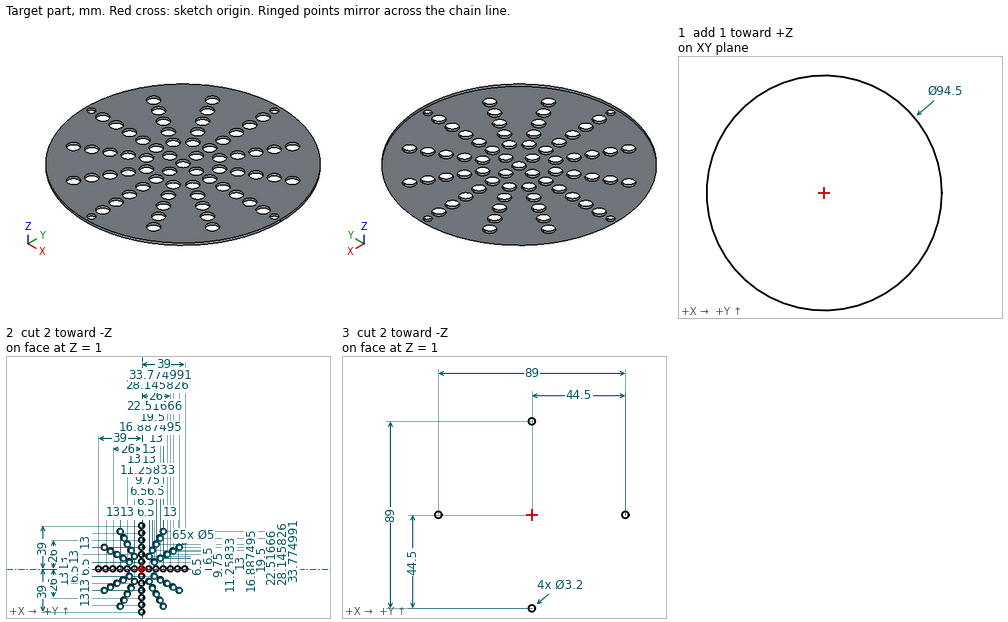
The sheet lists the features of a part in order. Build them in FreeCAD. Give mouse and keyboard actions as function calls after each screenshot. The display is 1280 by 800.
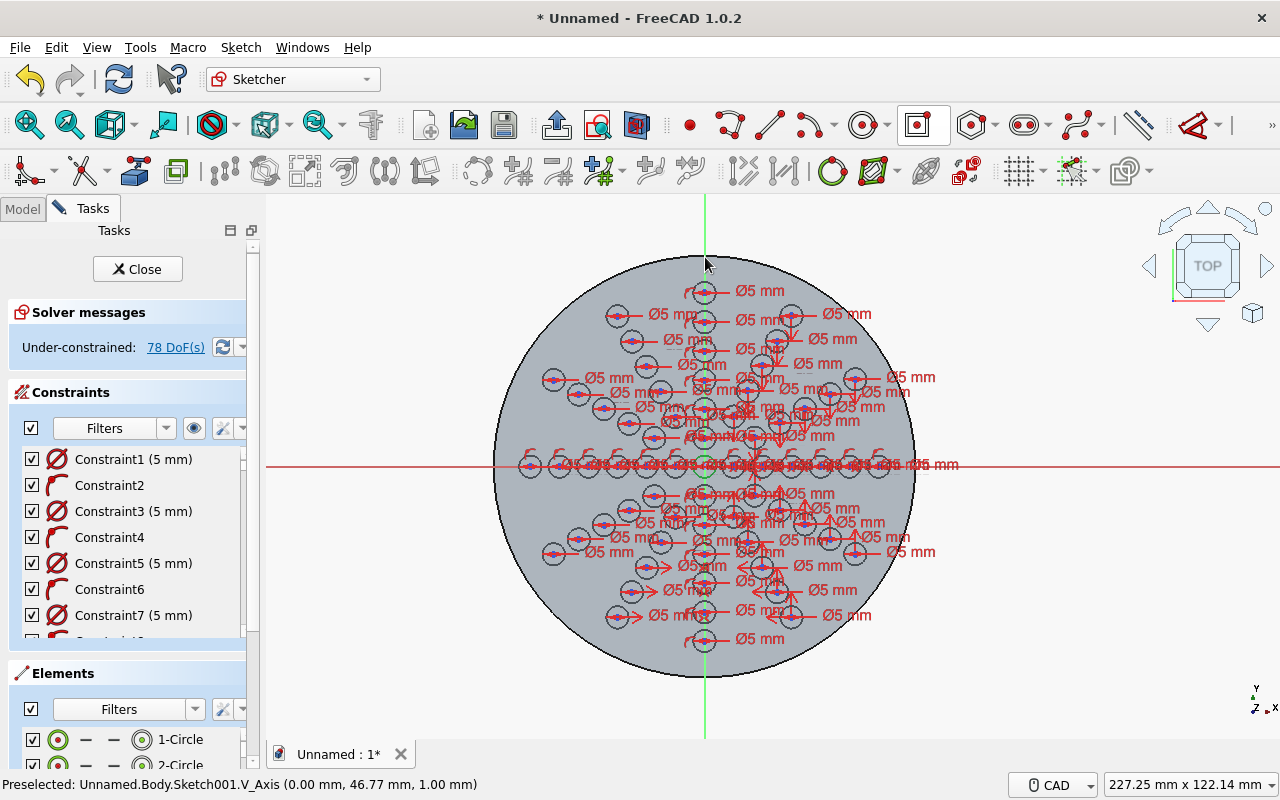
click(748, 542)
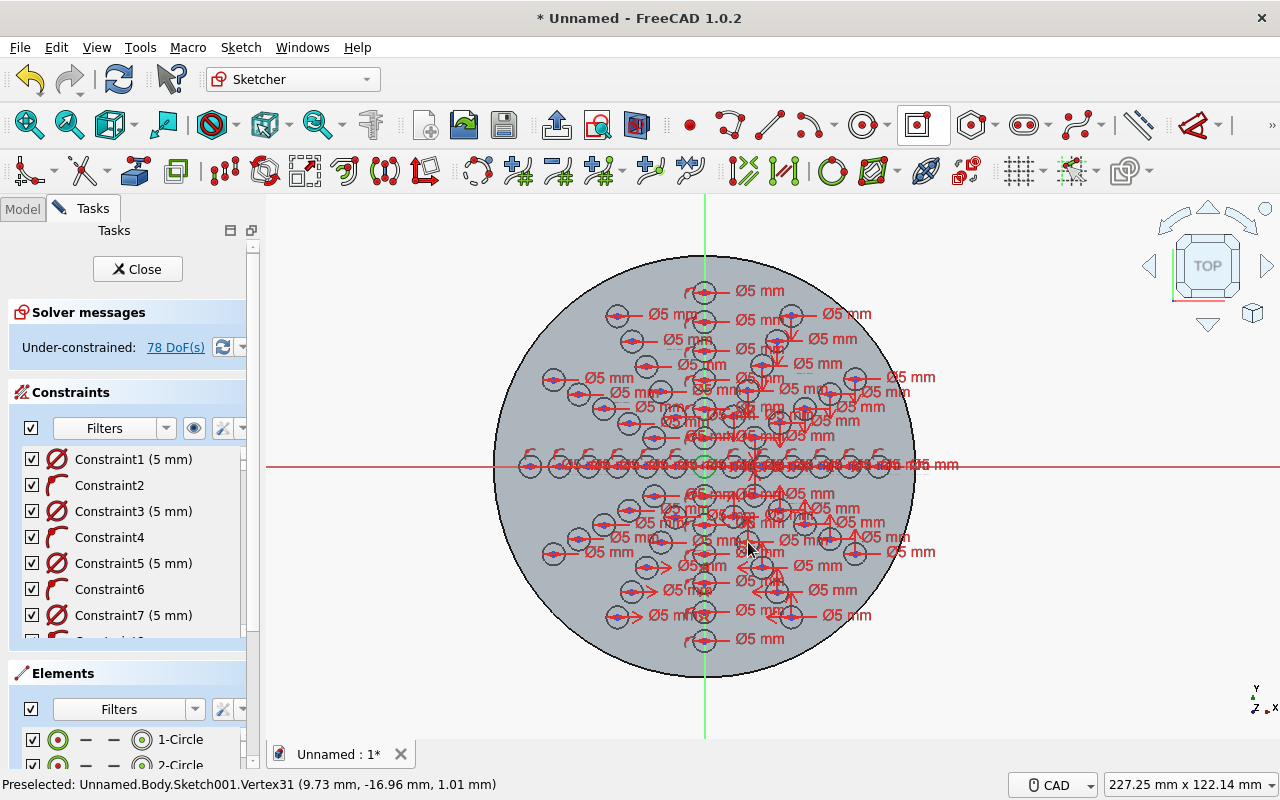
click(661, 543)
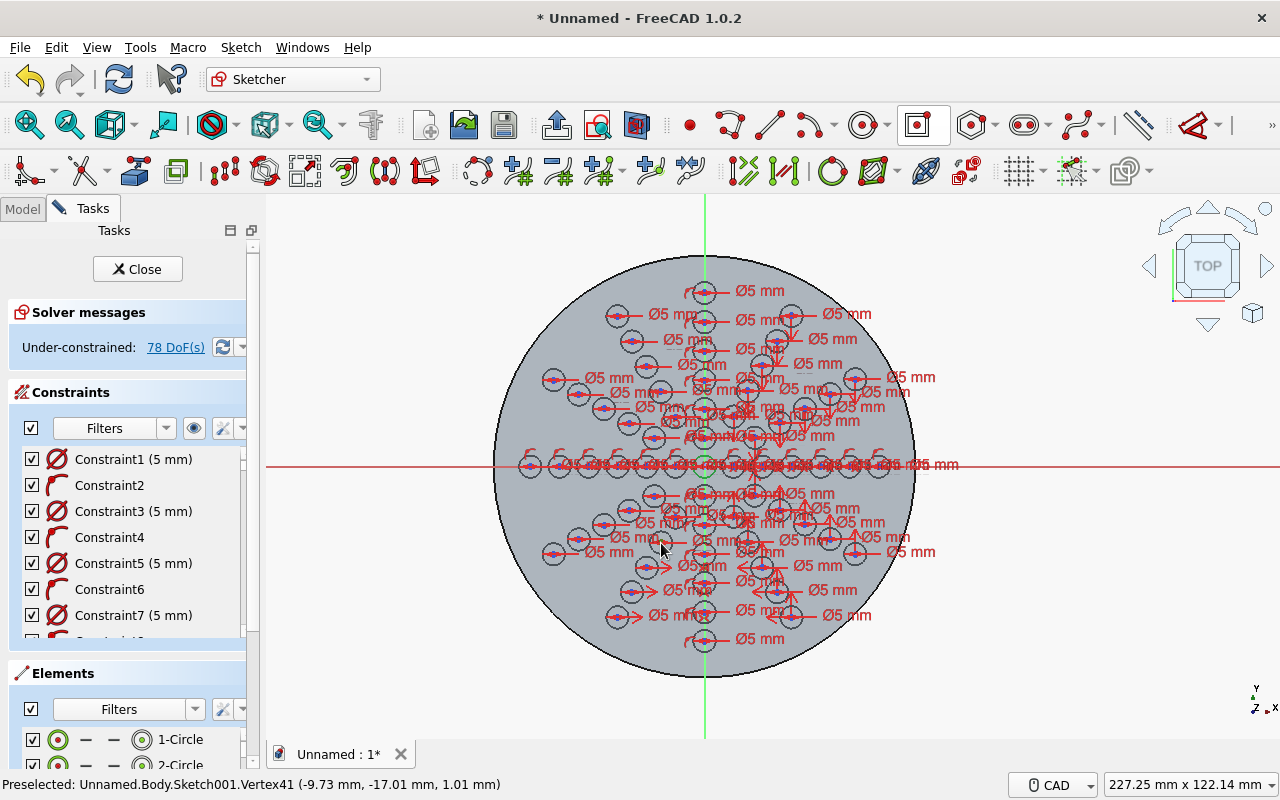
click(705, 257)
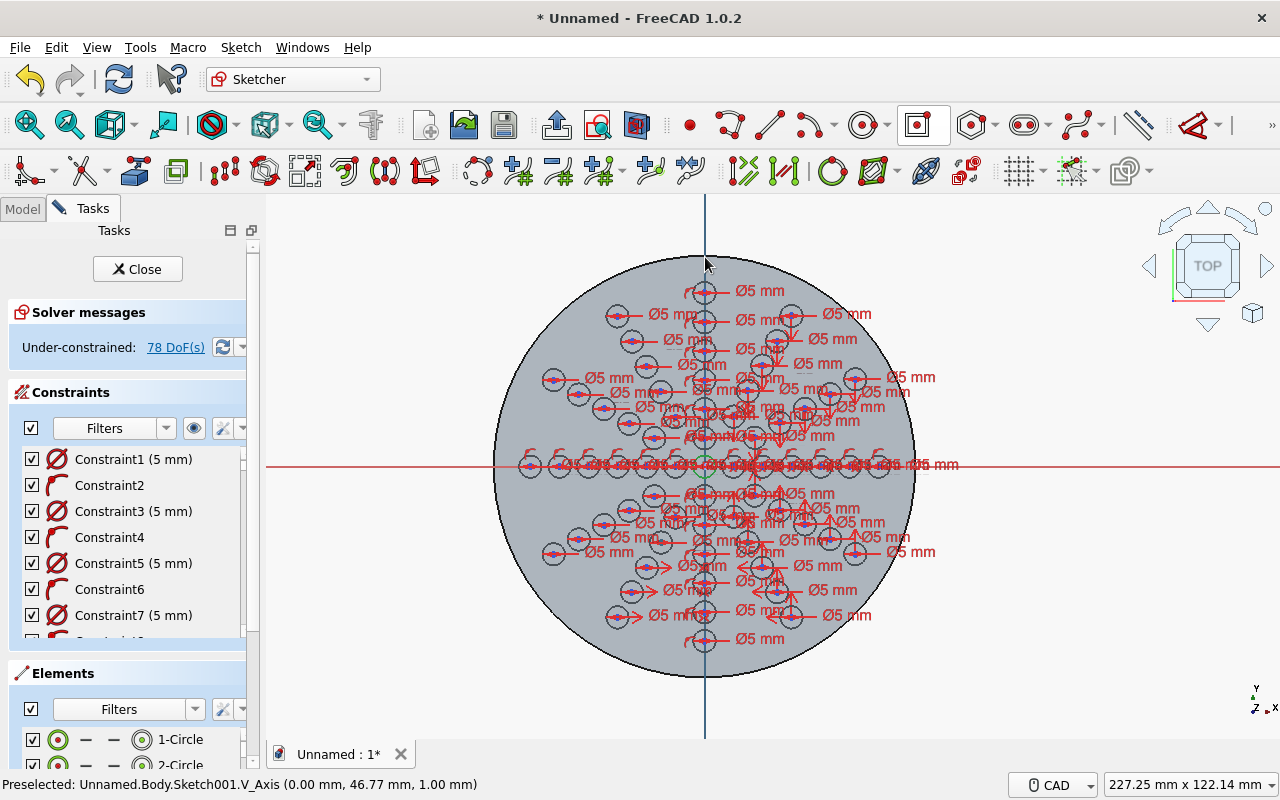
key(s)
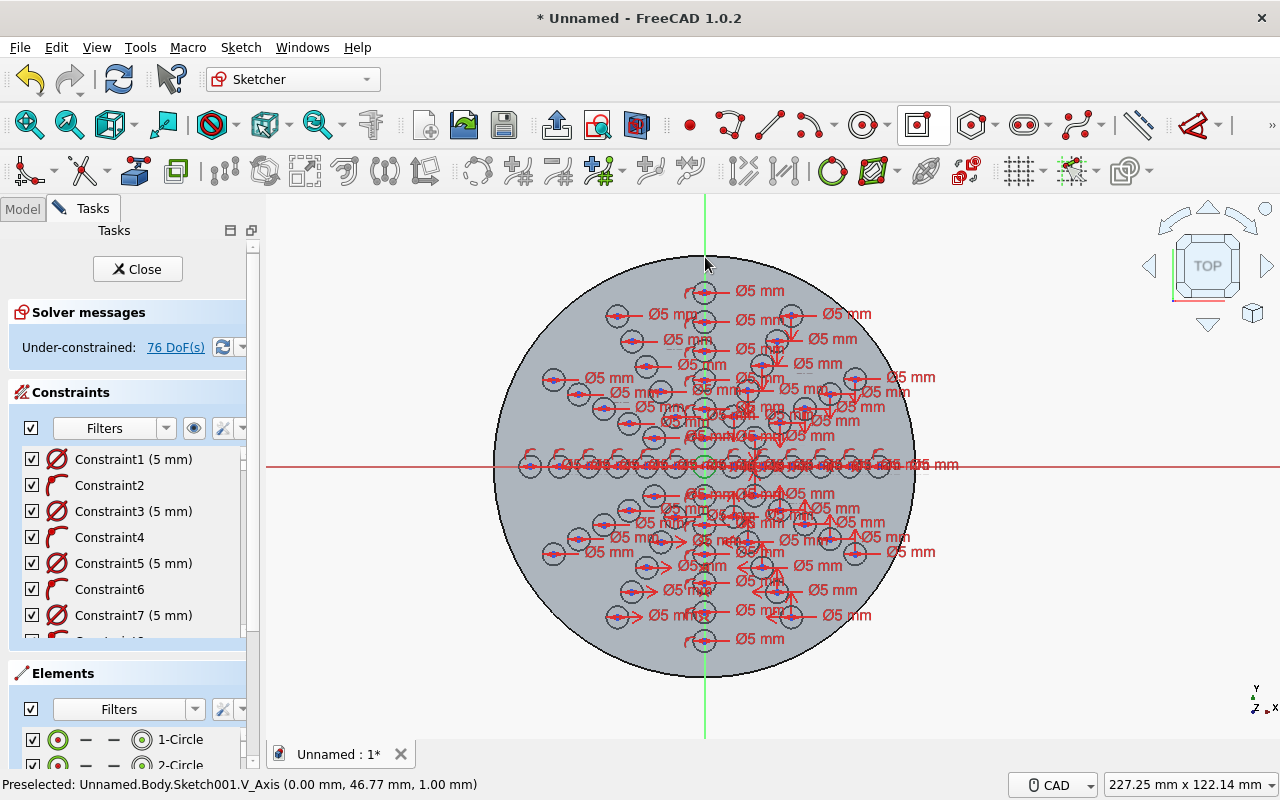
click(734, 517)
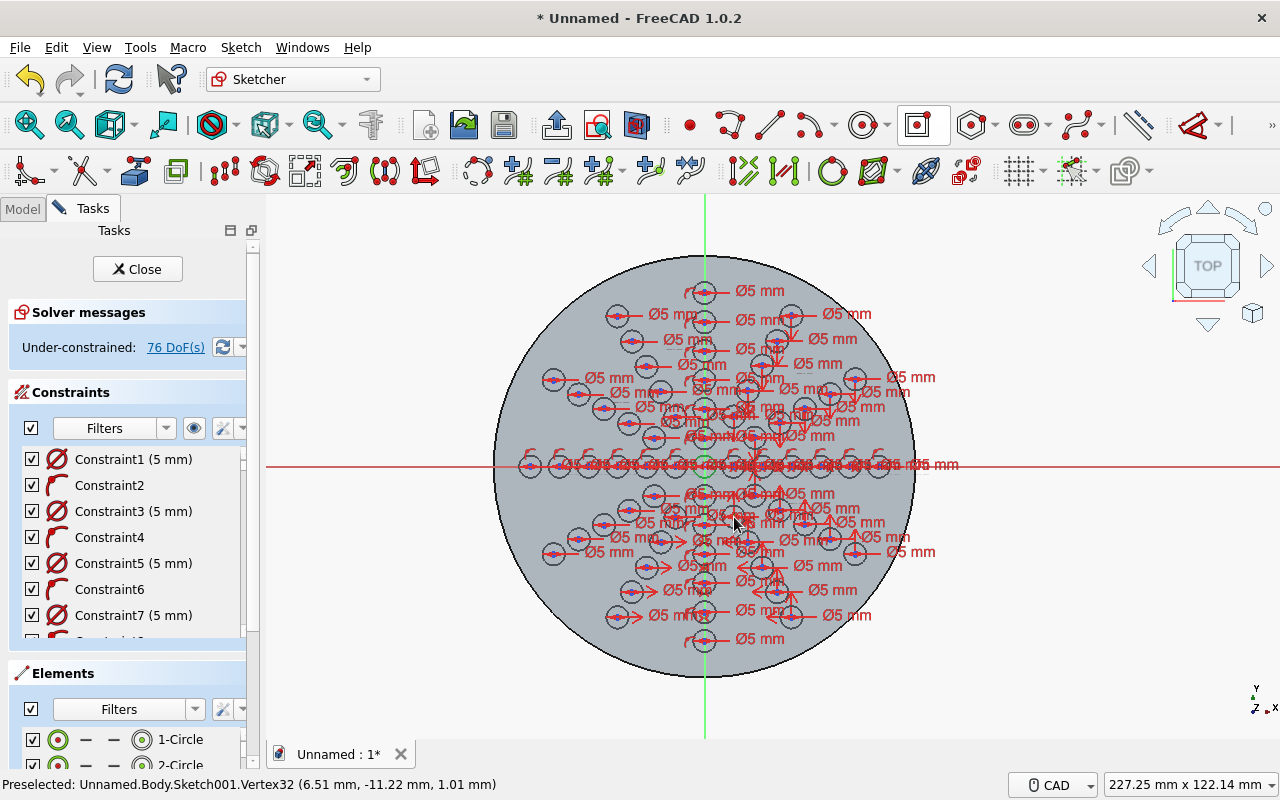
click(675, 517)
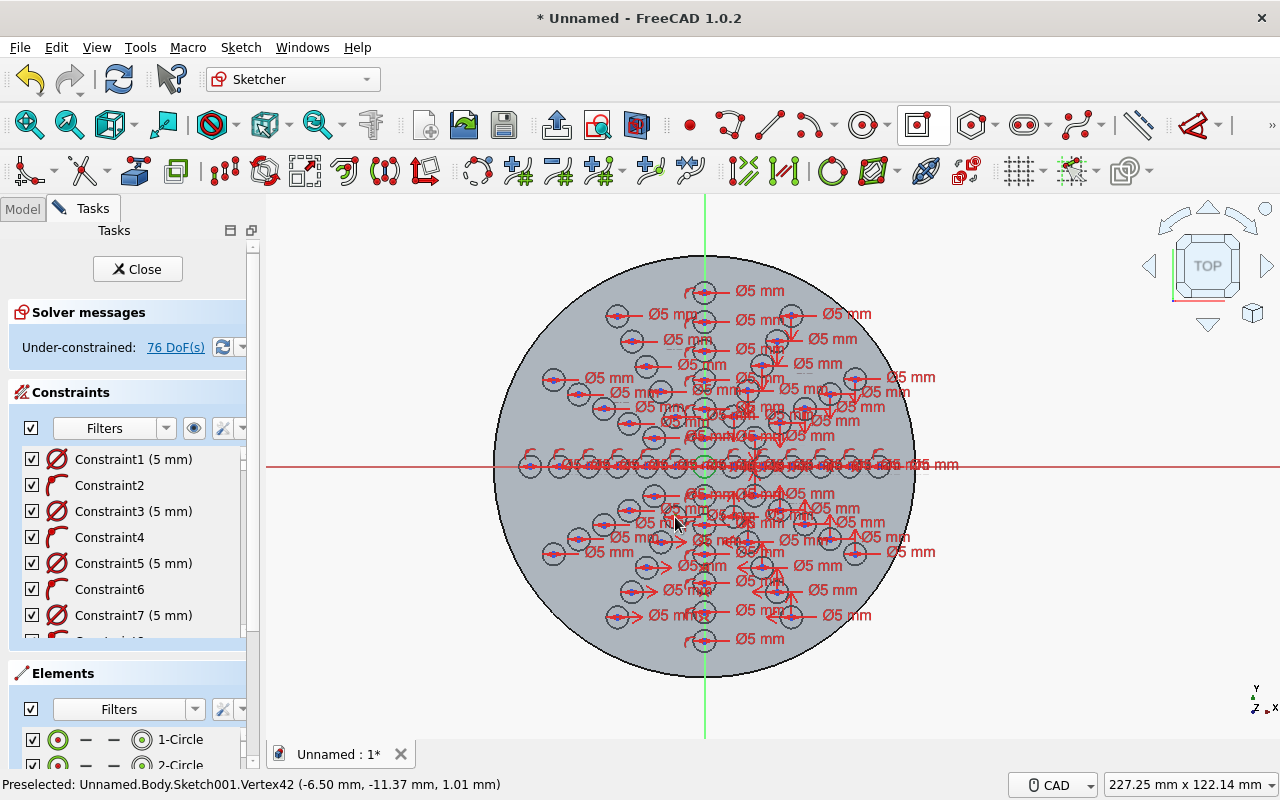
click(705, 257)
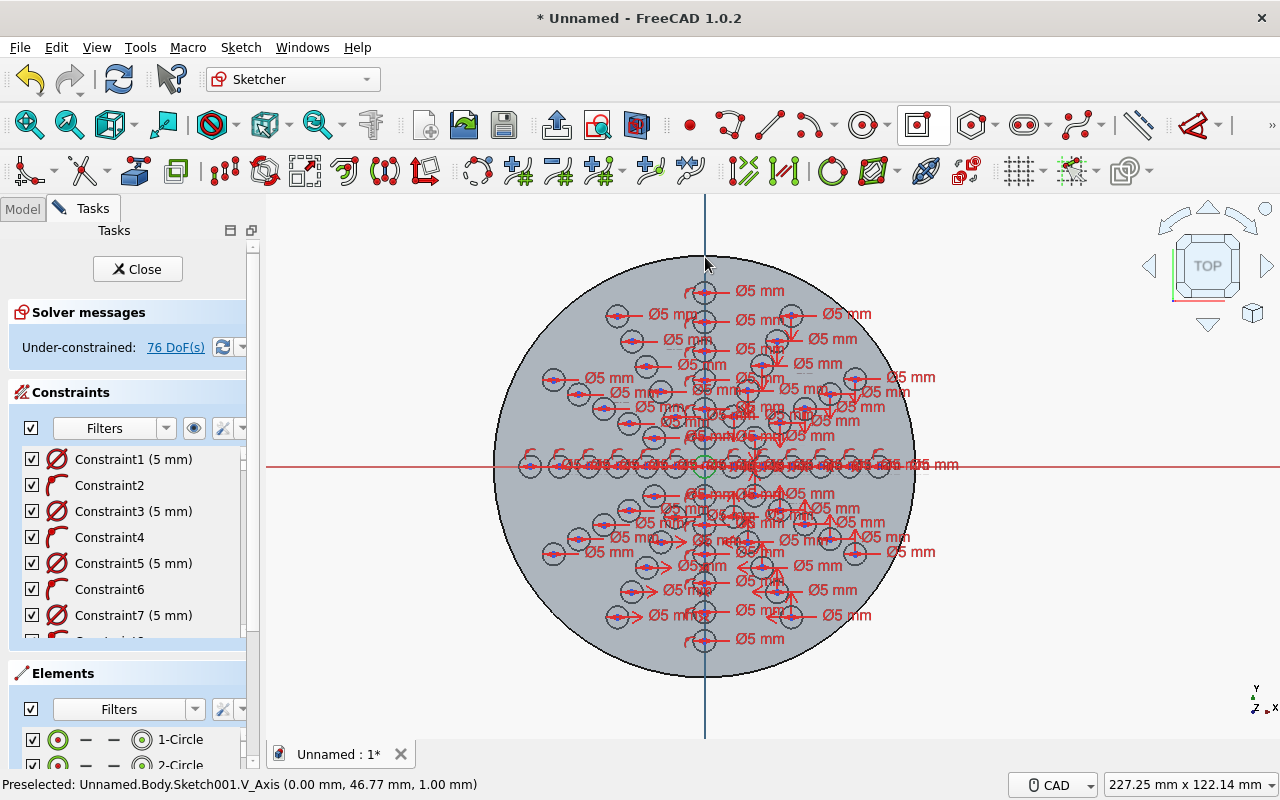
key(s)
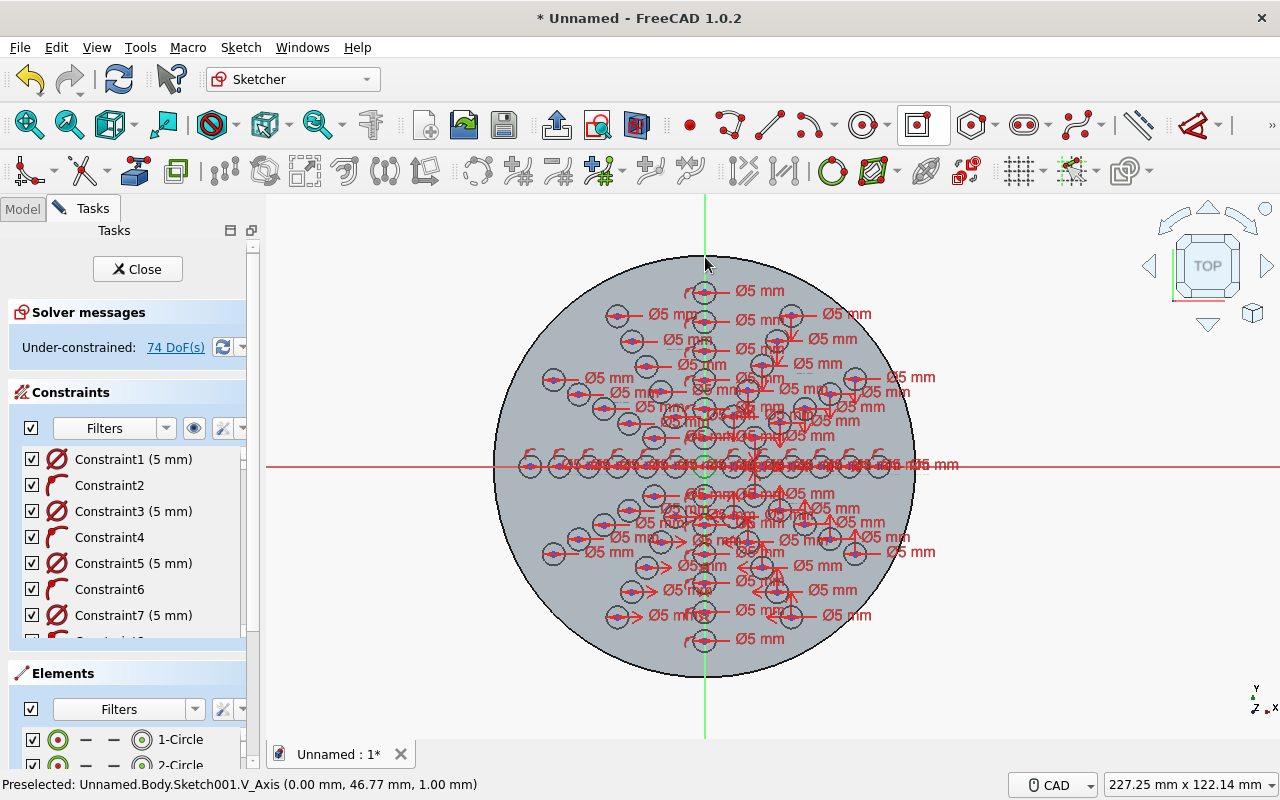
click(855, 554)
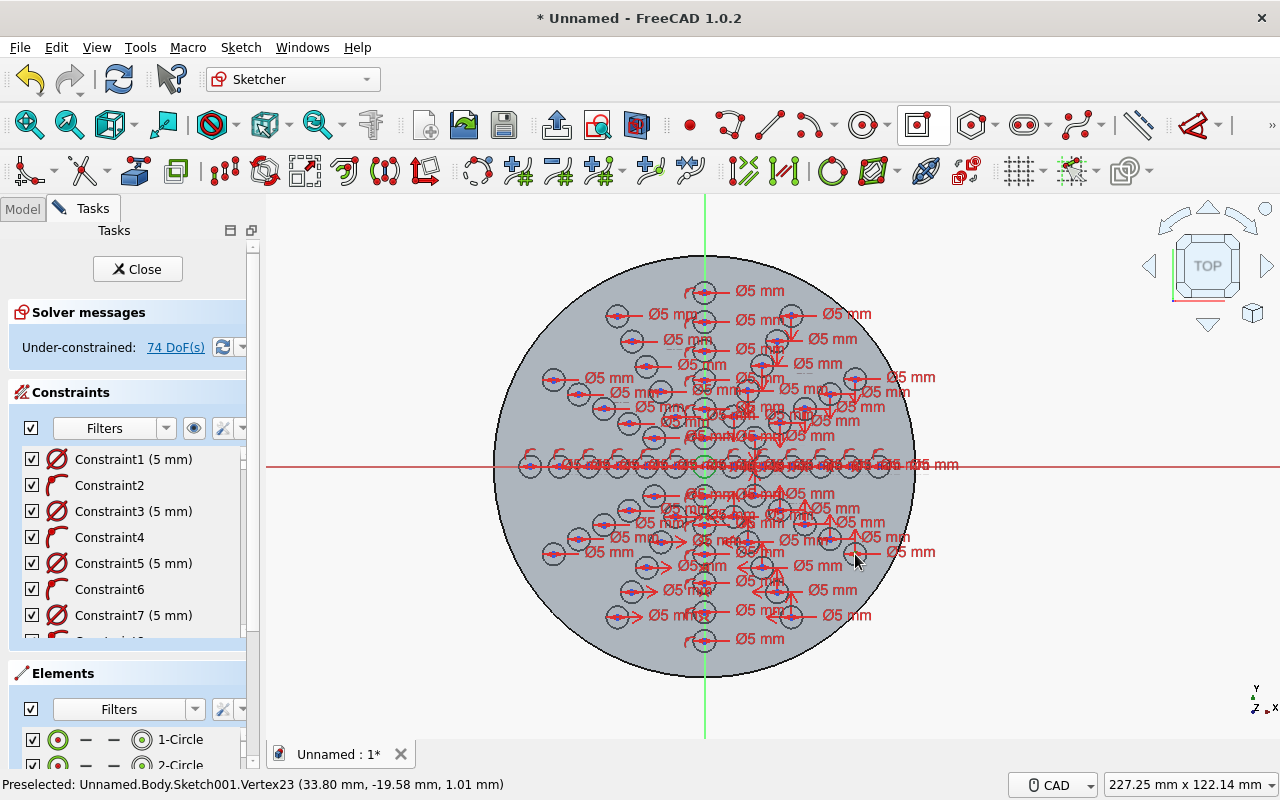
click(554, 554)